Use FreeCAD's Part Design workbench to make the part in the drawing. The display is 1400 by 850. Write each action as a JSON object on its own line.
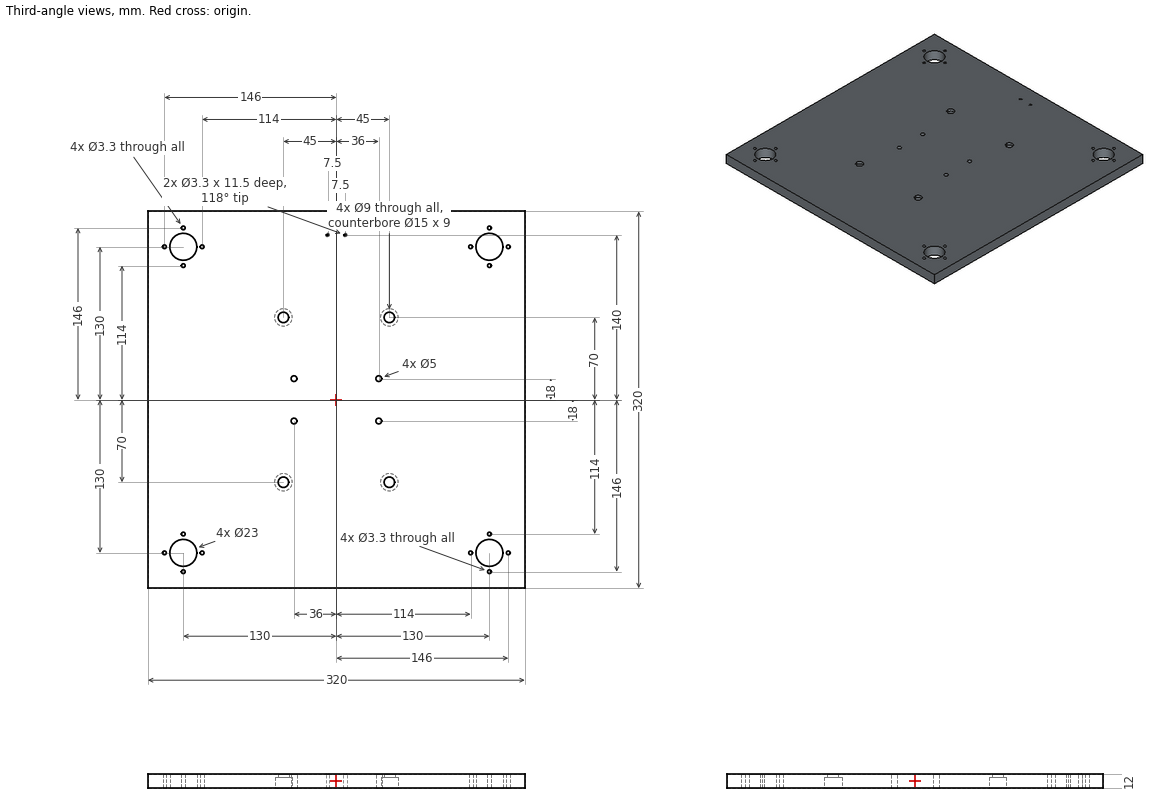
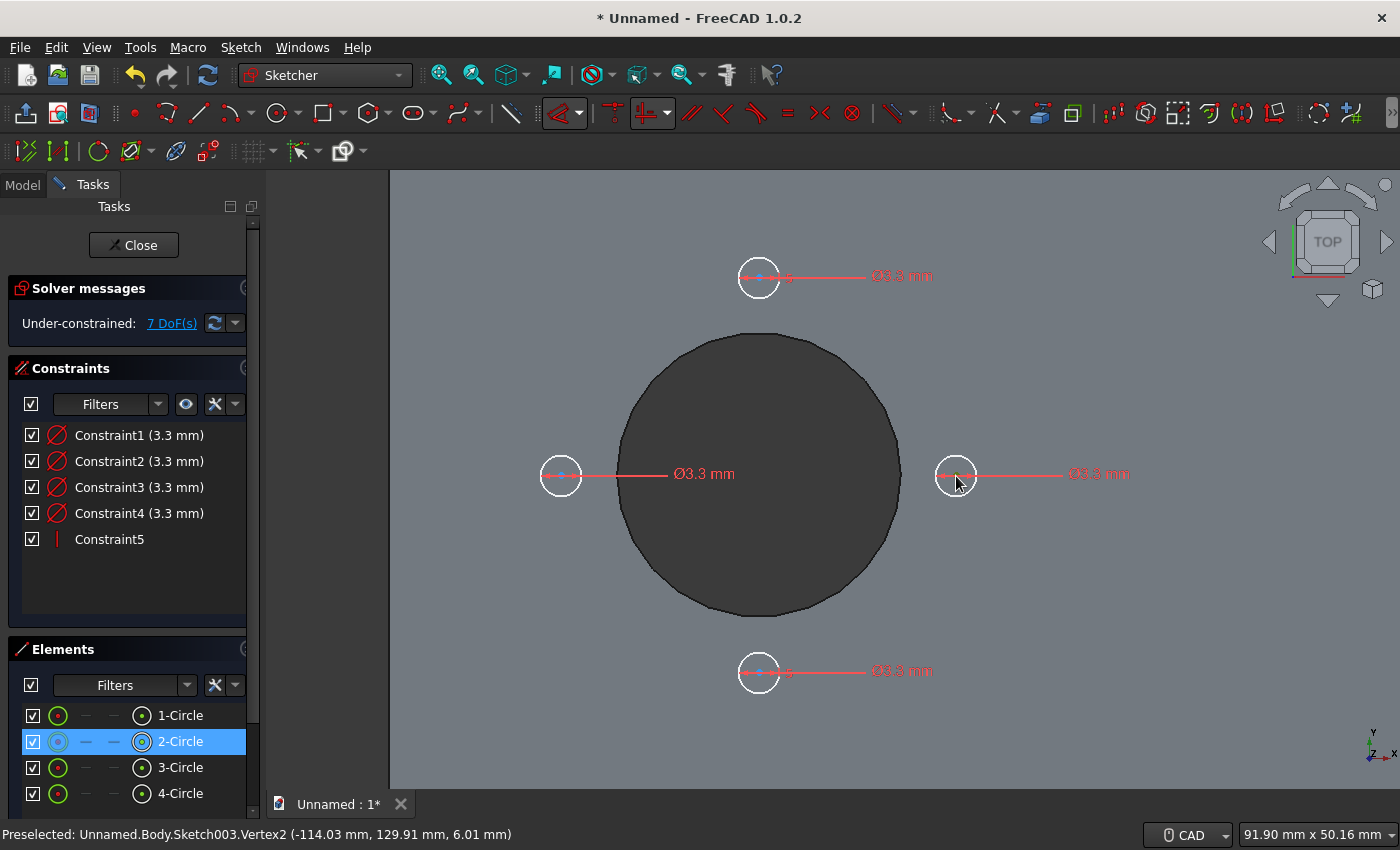
{"action": "left_click", "coordinate": [561, 476]}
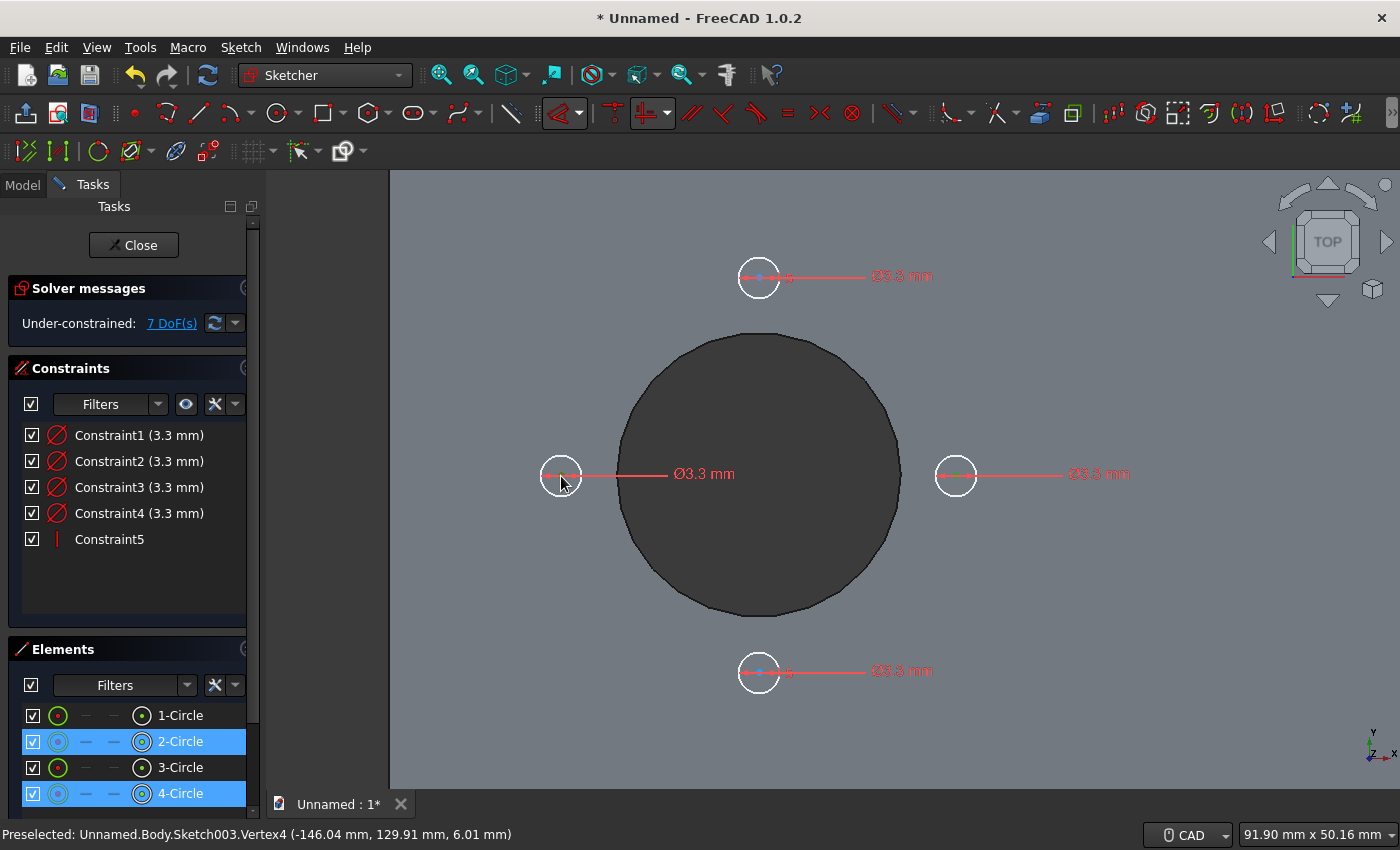
{"action": "key", "text": "h"}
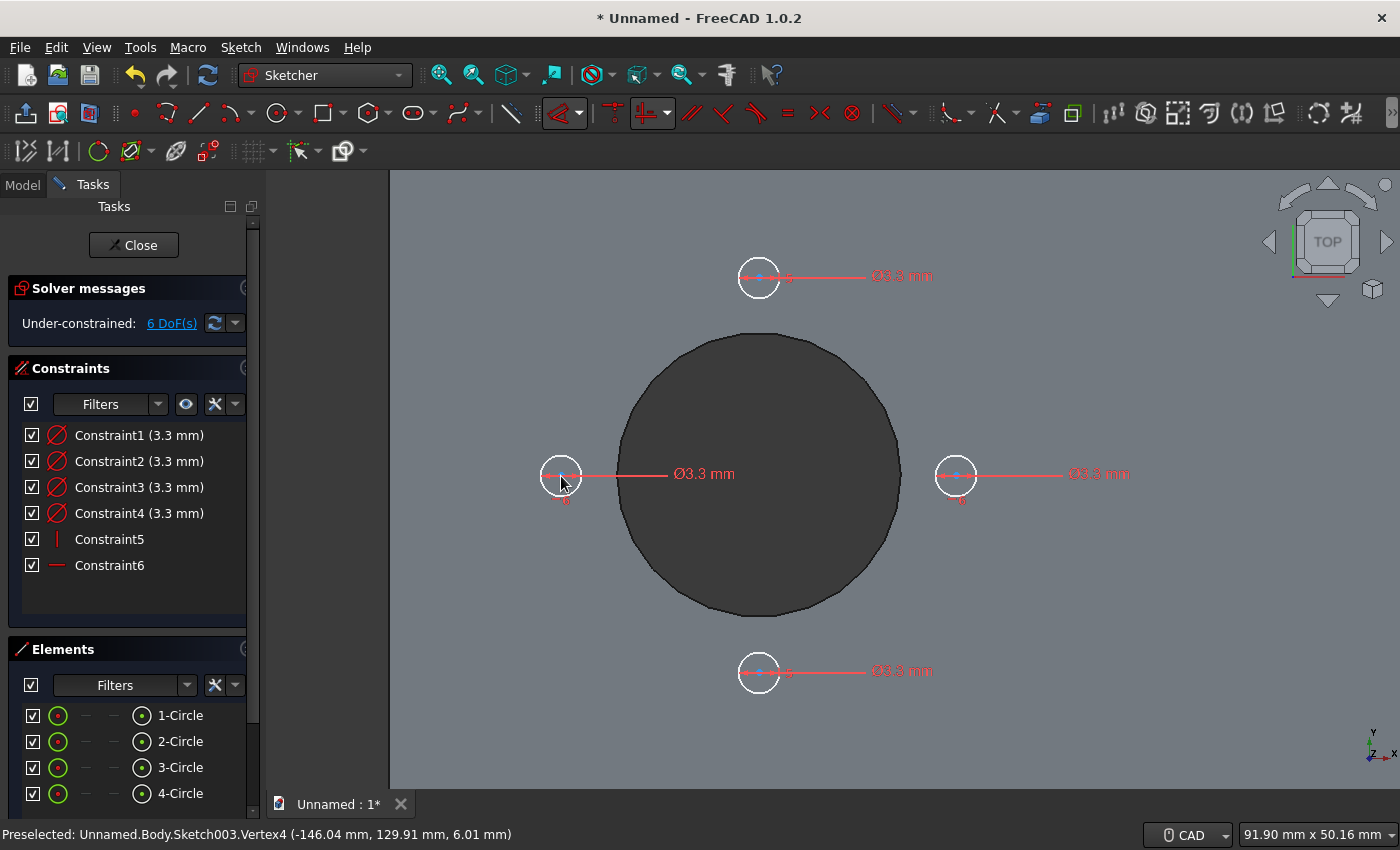
{"action": "left_click", "coordinate": [759, 278]}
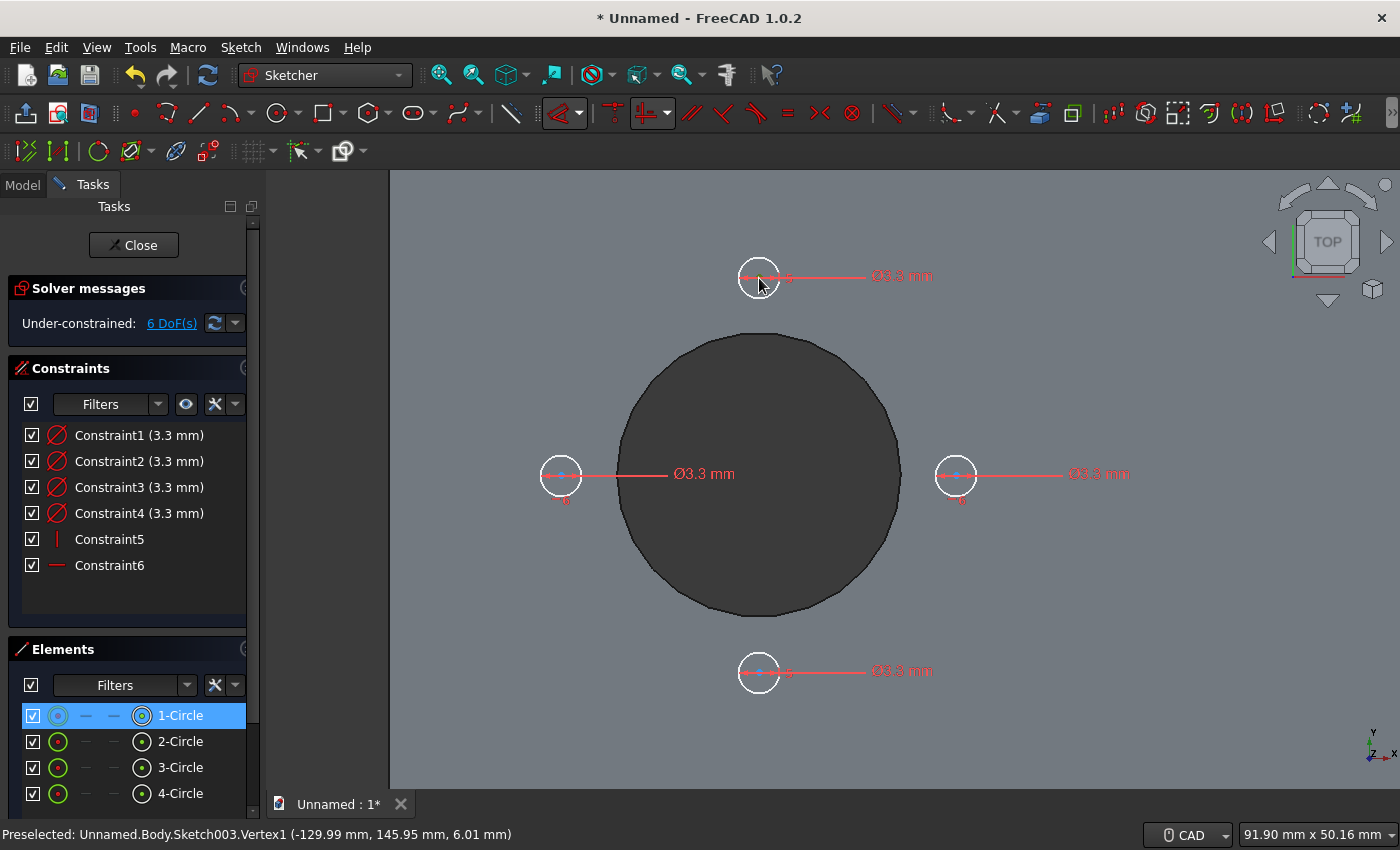
{"action": "key", "text": "l"}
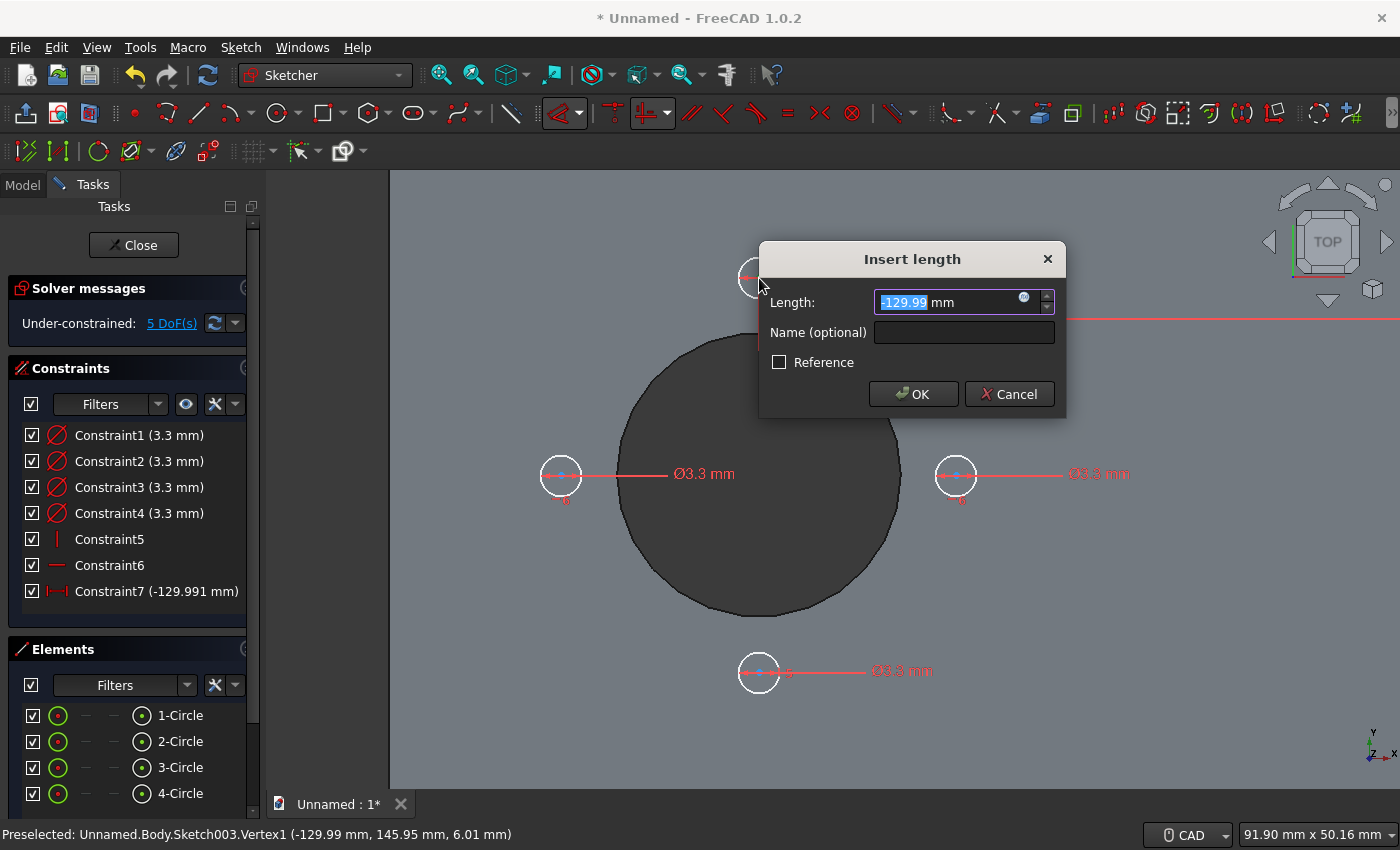
{"action": "type", "text": "-130"}
{"action": "key", "text": "Return"}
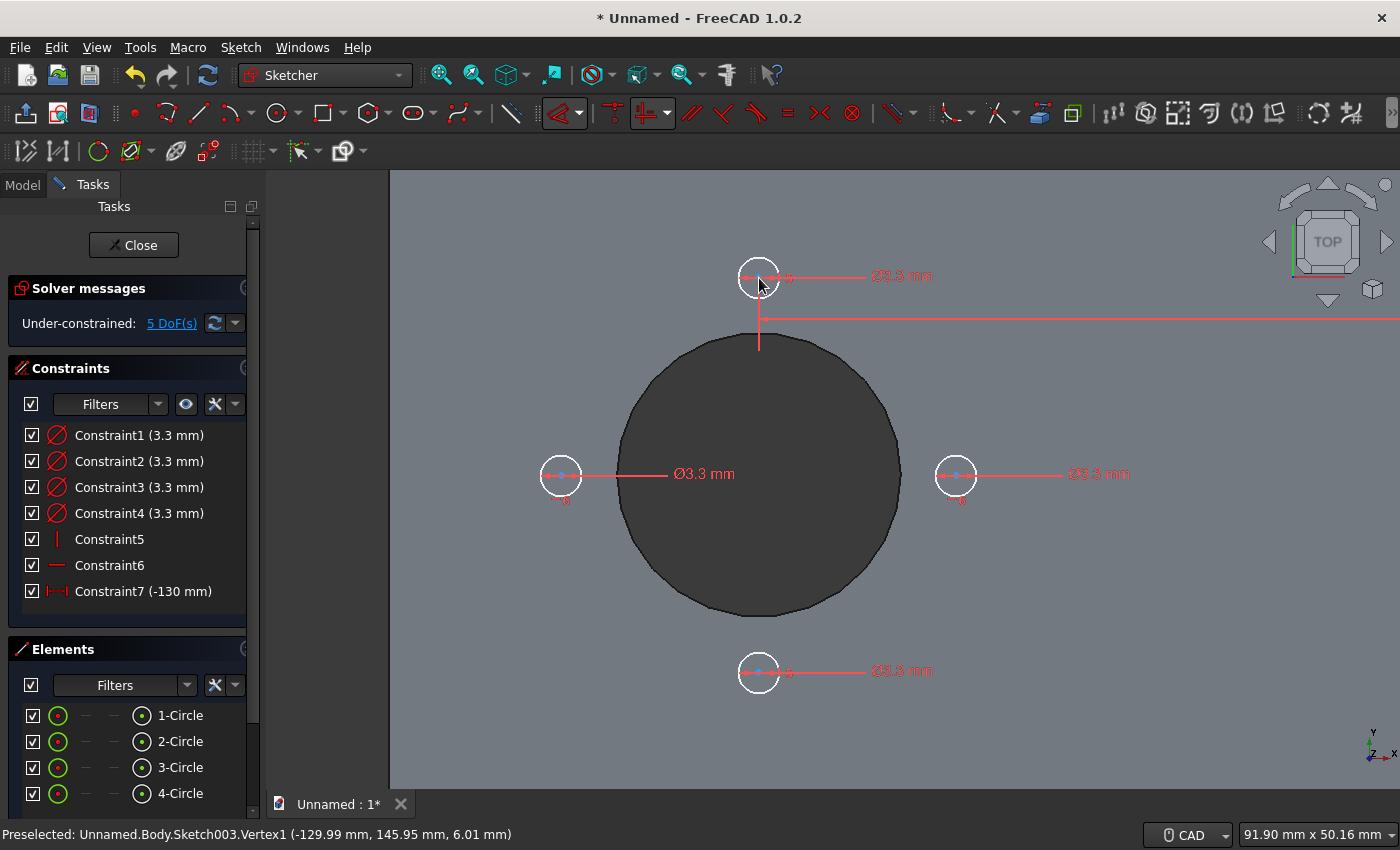
{"action": "left_click", "coordinate": [759, 278]}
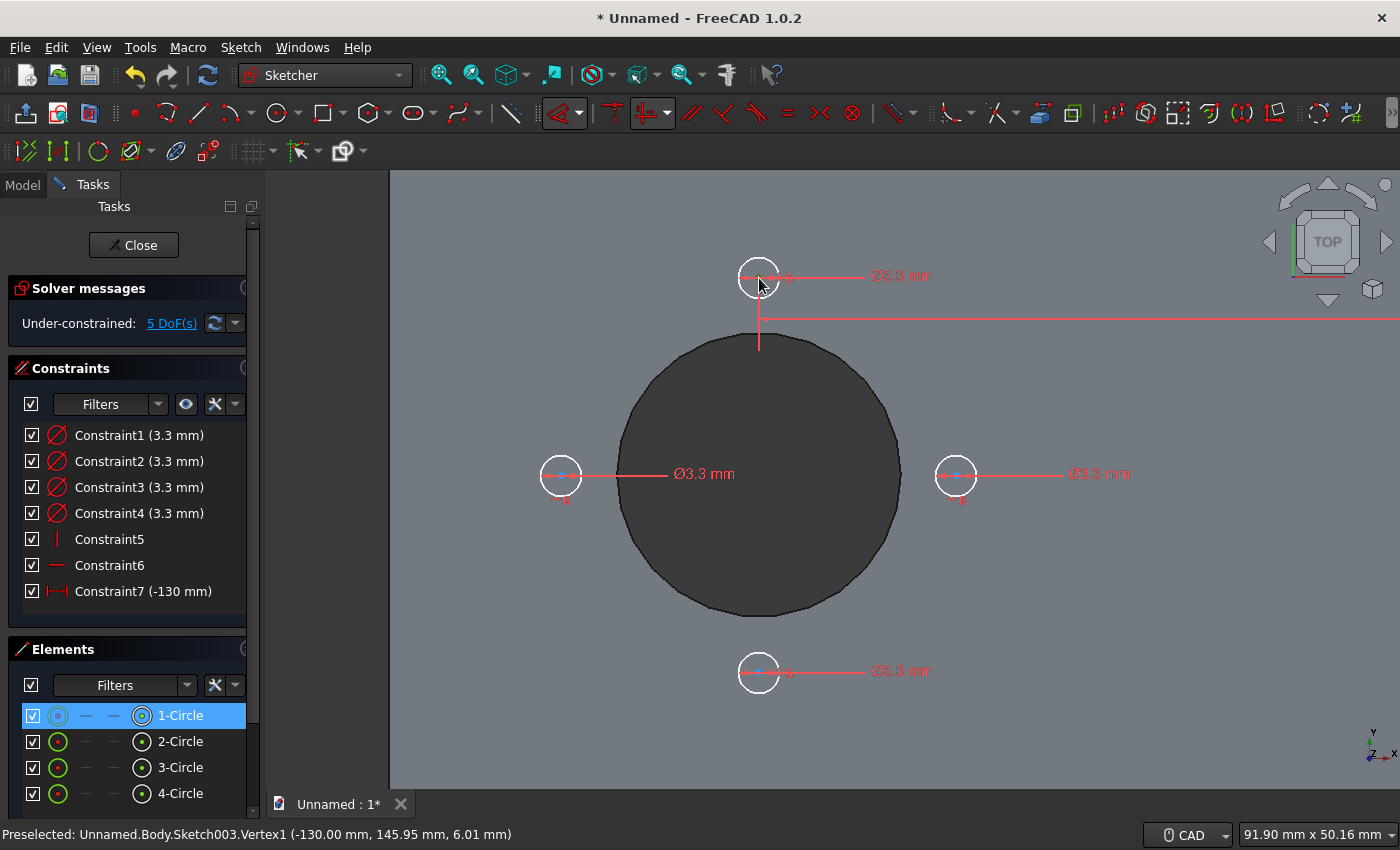
{"action": "key", "text": "i"}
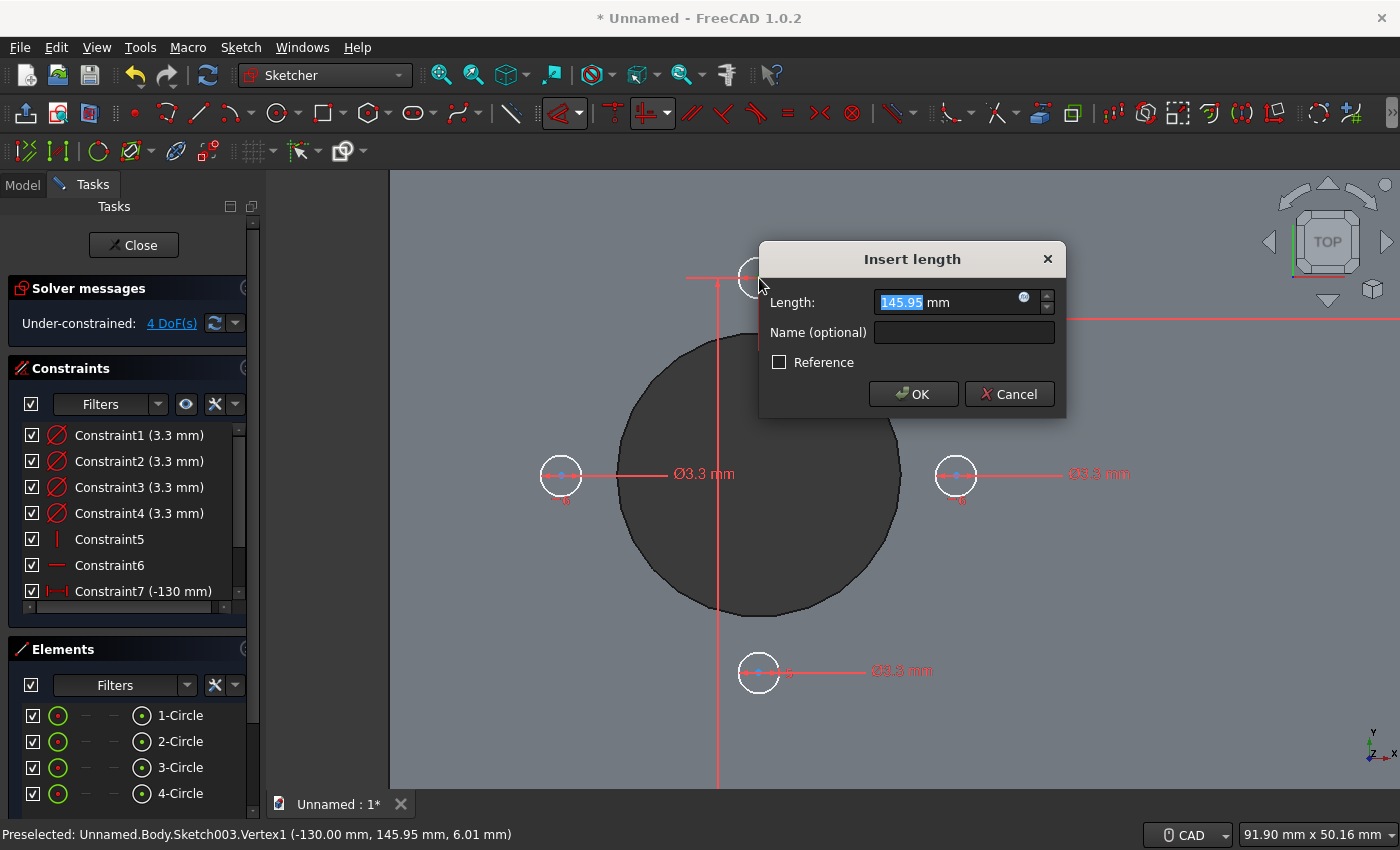
{"action": "type", "text": "146"}
{"action": "key", "text": "Return"}